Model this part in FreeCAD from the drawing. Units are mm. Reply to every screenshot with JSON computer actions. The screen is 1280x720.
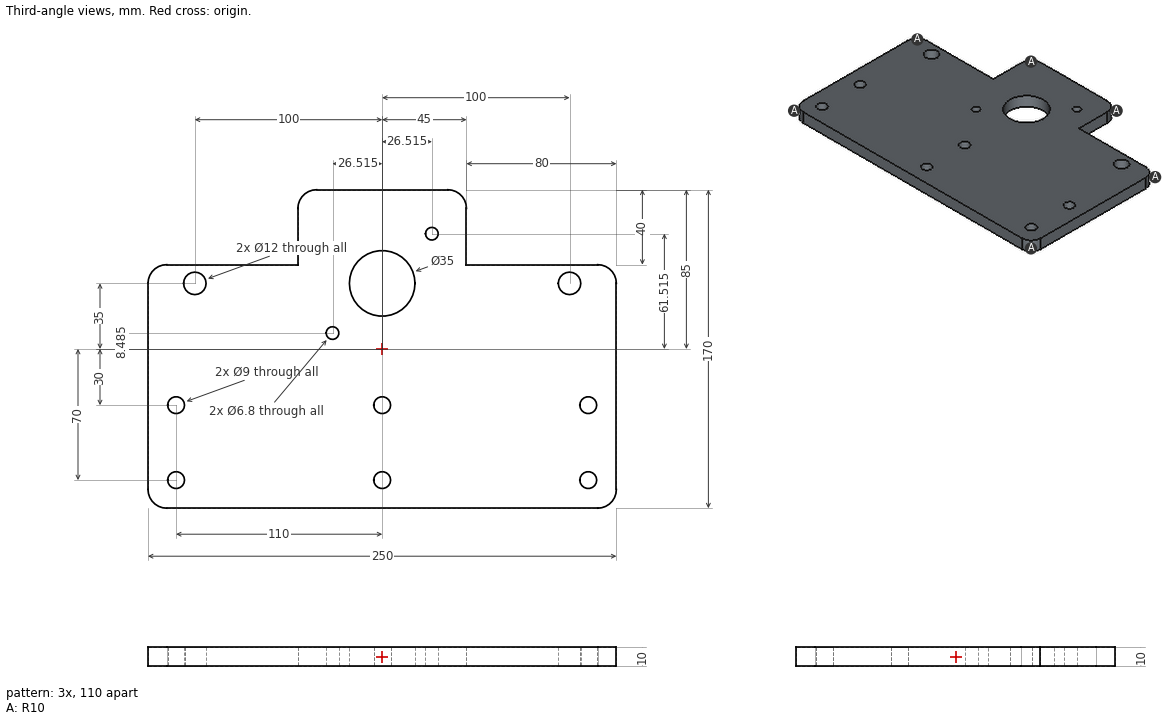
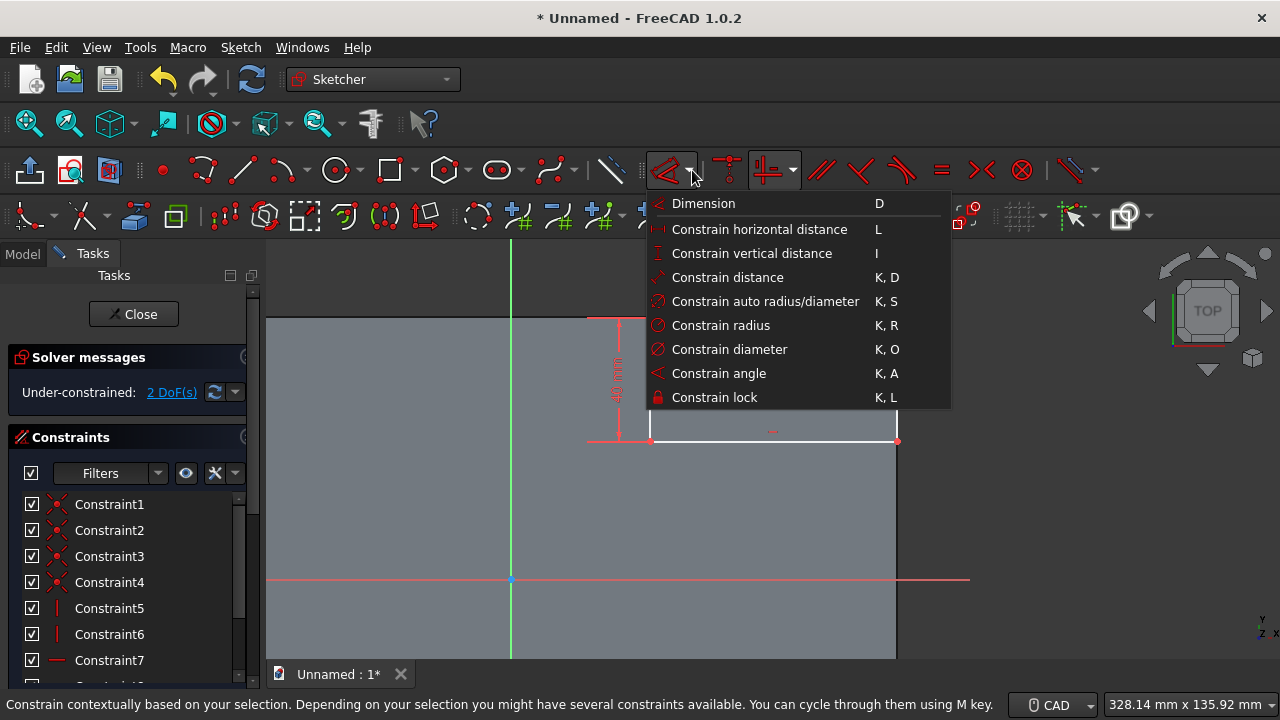
{"action": "left_click", "coordinate": [799, 229]}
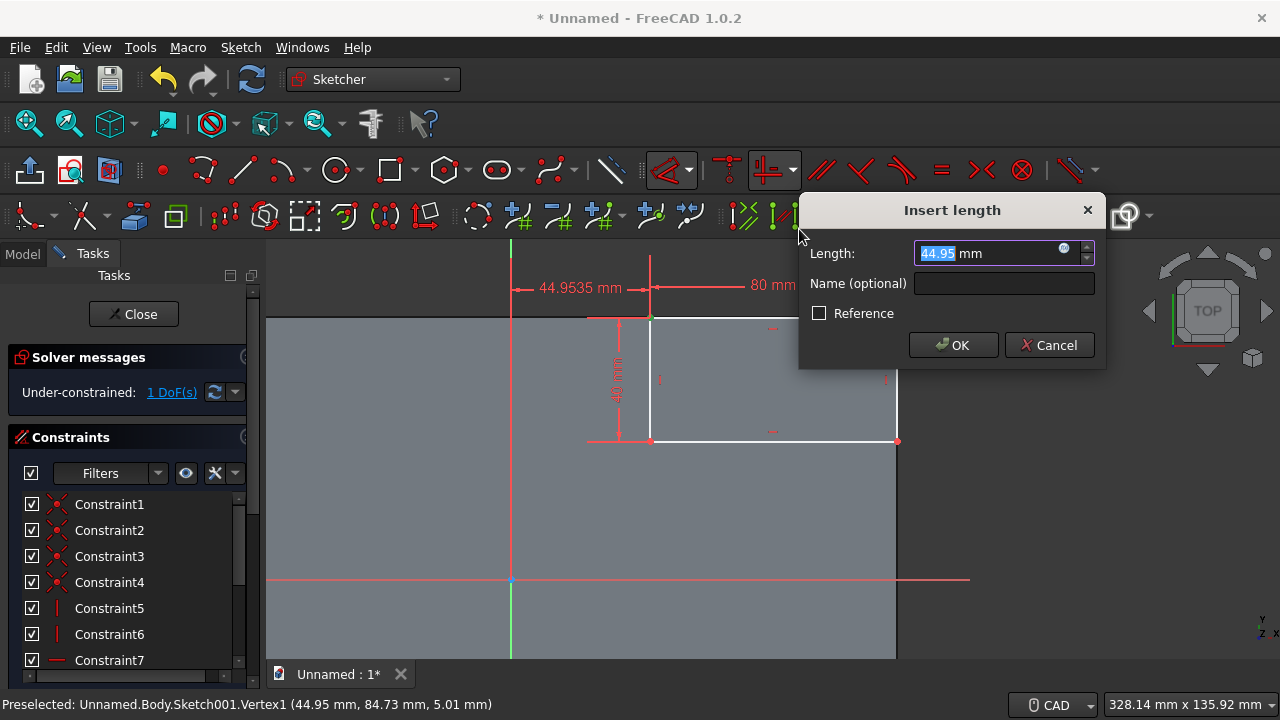
{"action": "type", "text": "45"}
{"action": "key", "text": "Return"}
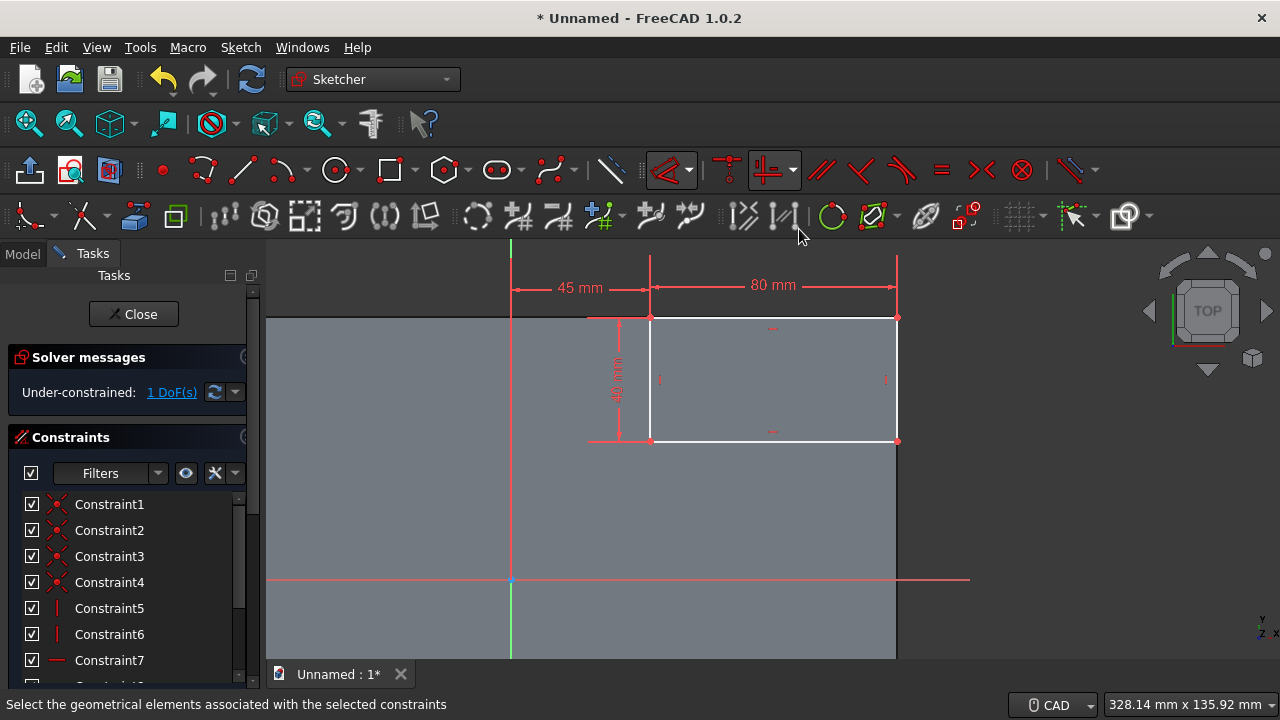
{"action": "left_click", "coordinate": [650, 318]}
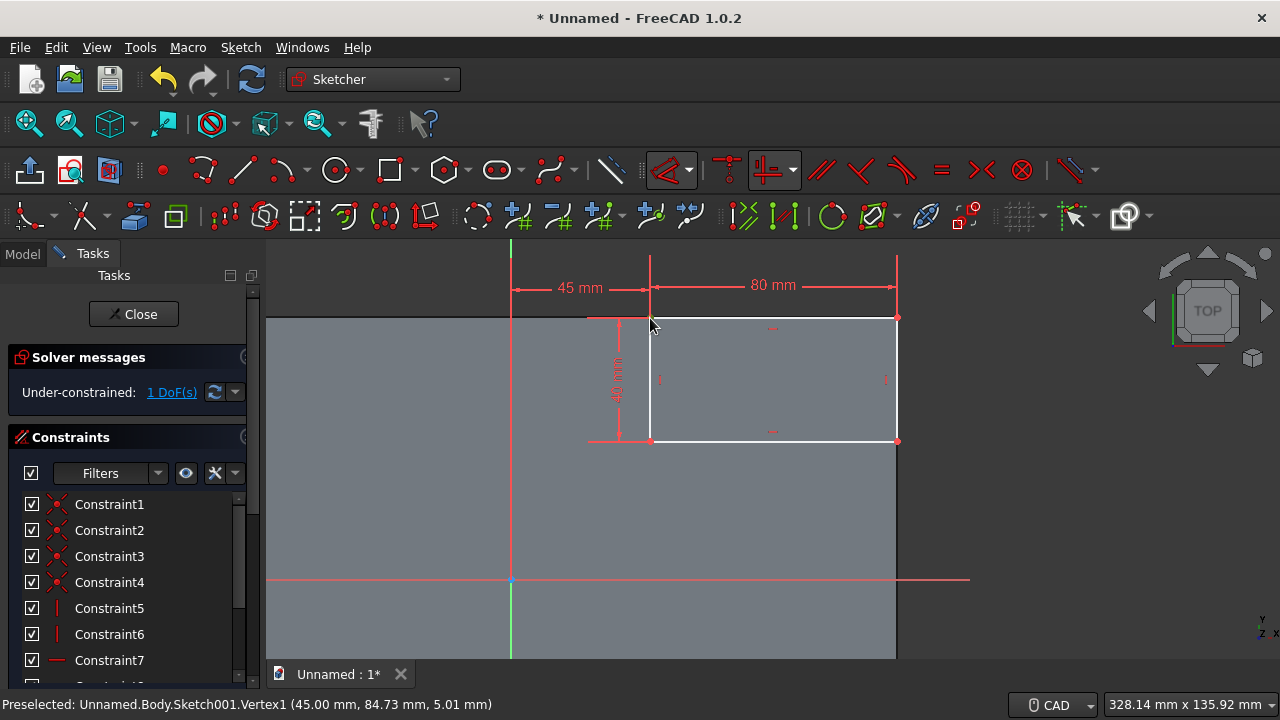
{"action": "left_click", "coordinate": [692, 170]}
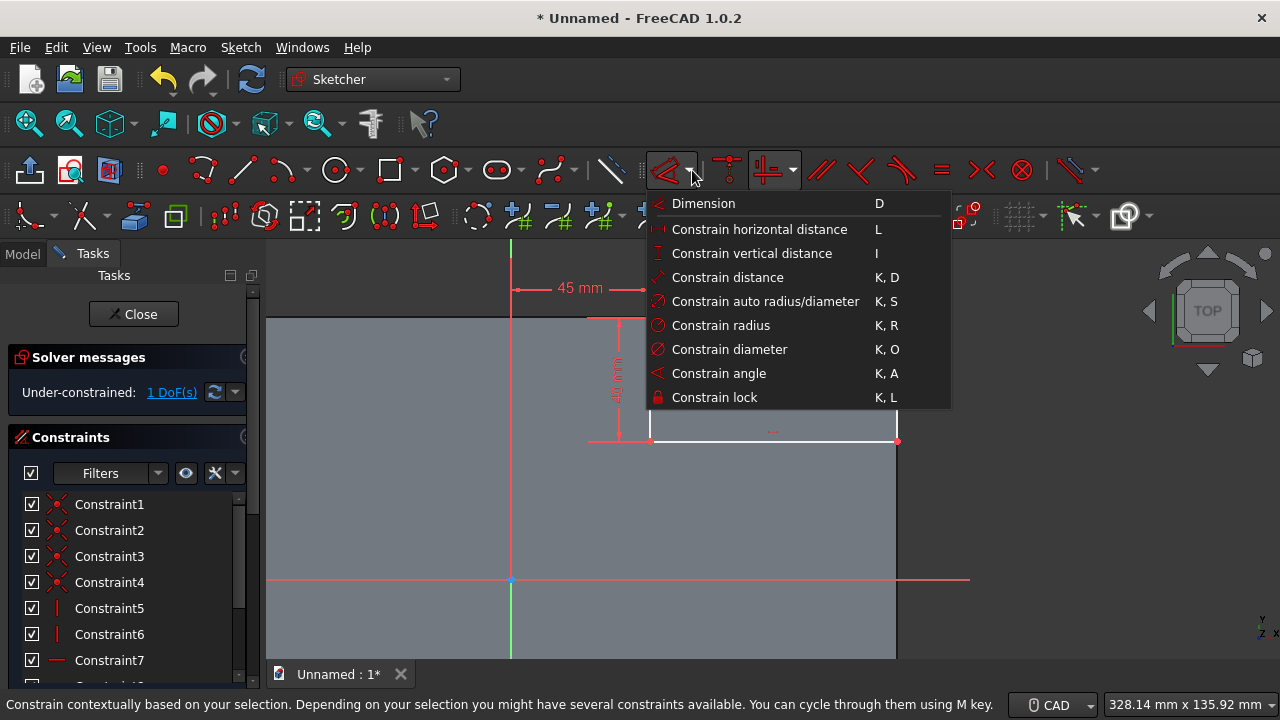
{"action": "left_click", "coordinate": [799, 253]}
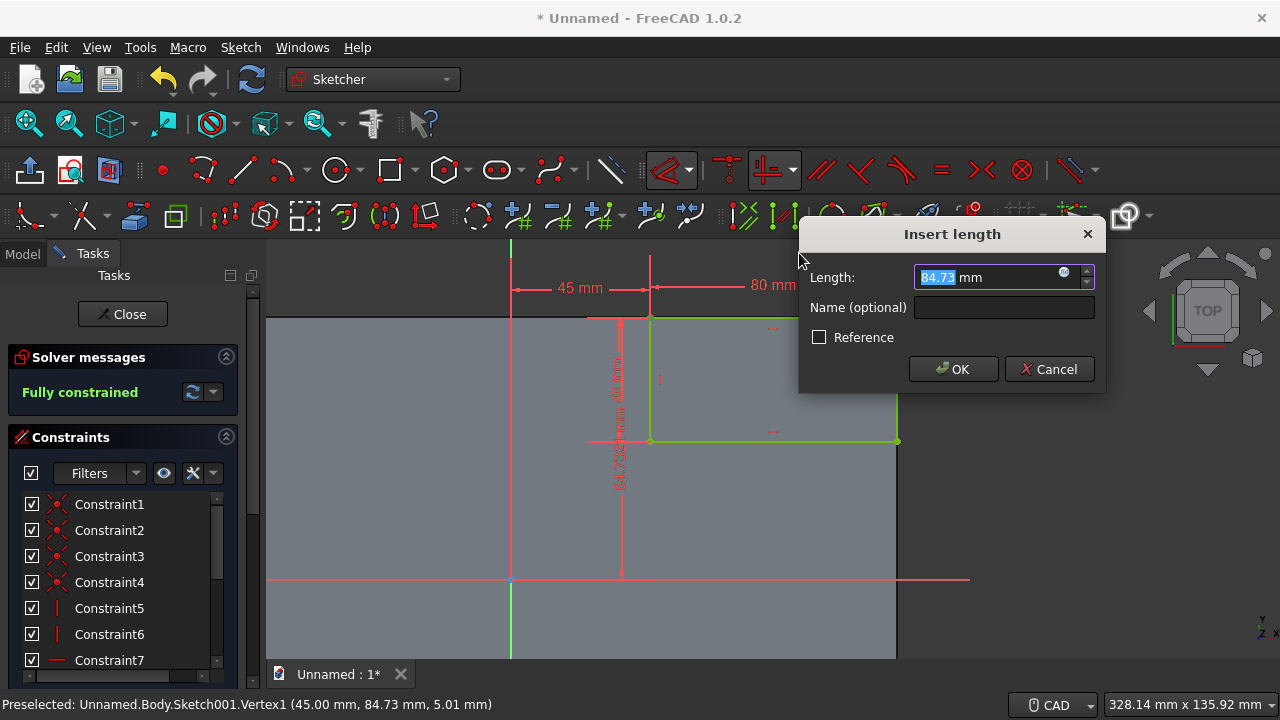
{"action": "type", "text": "85"}
{"action": "key", "text": "Return"}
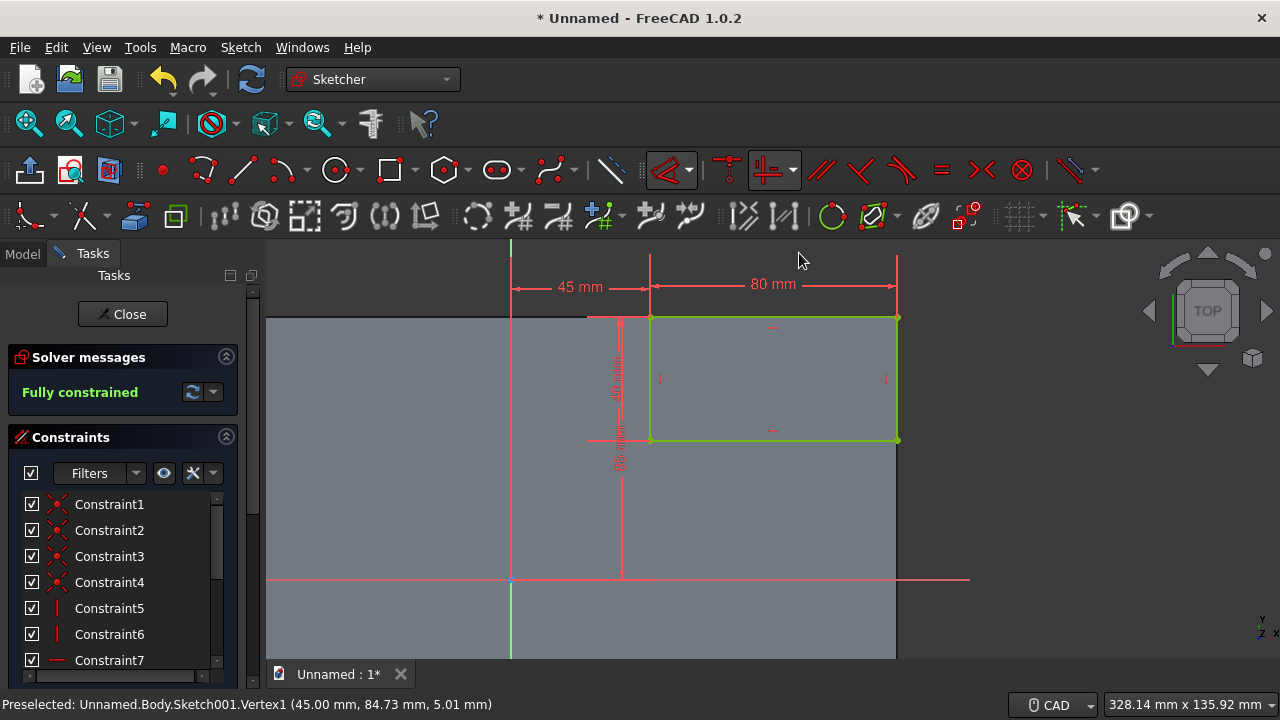
{"action": "left_click", "coordinate": [123, 314]}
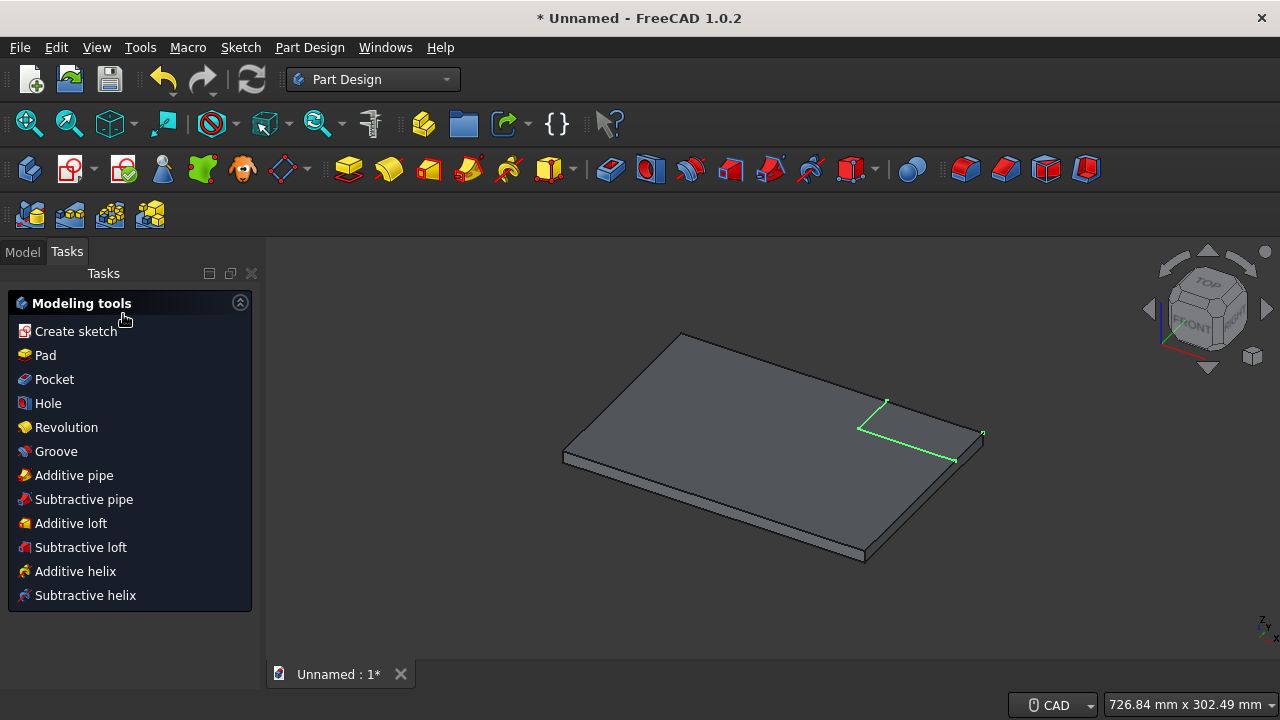
{"action": "left_click", "coordinate": [612, 170]}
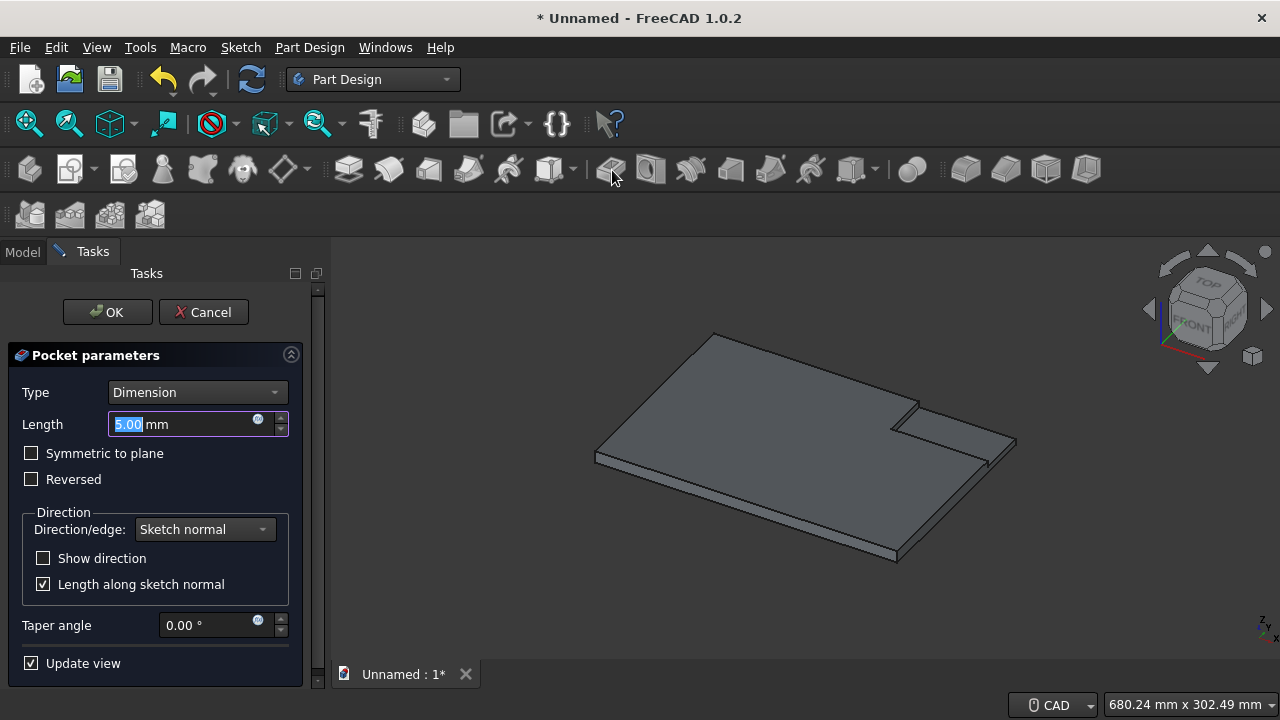
{"action": "type", "text": "10"}
{"action": "key", "text": "Tab"}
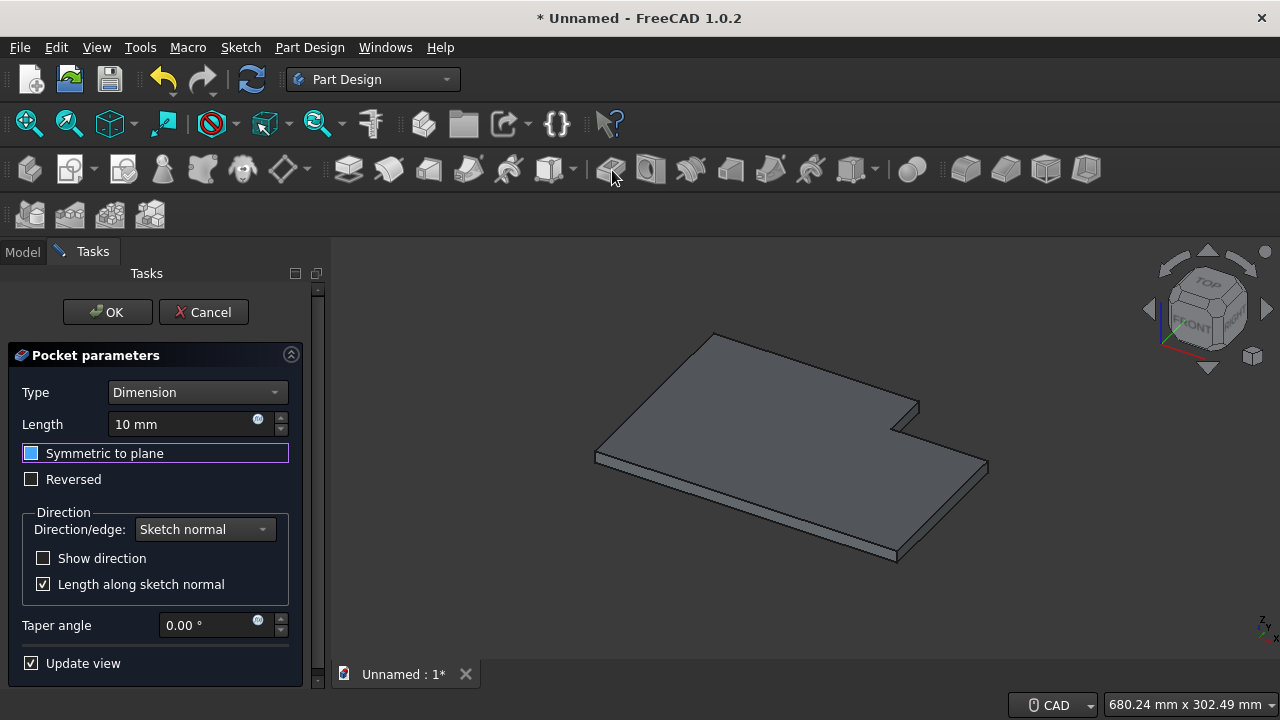
{"action": "left_click", "coordinate": [108, 312]}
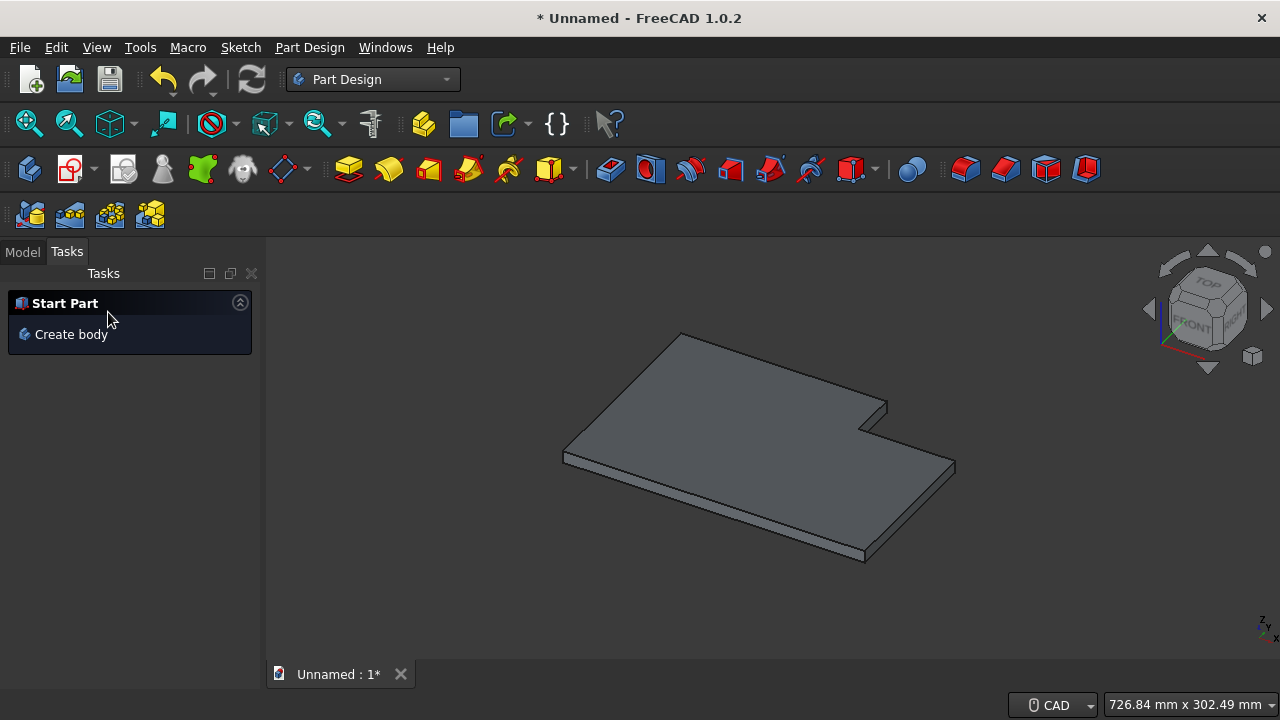
{"action": "left_click", "coordinate": [23, 251]}